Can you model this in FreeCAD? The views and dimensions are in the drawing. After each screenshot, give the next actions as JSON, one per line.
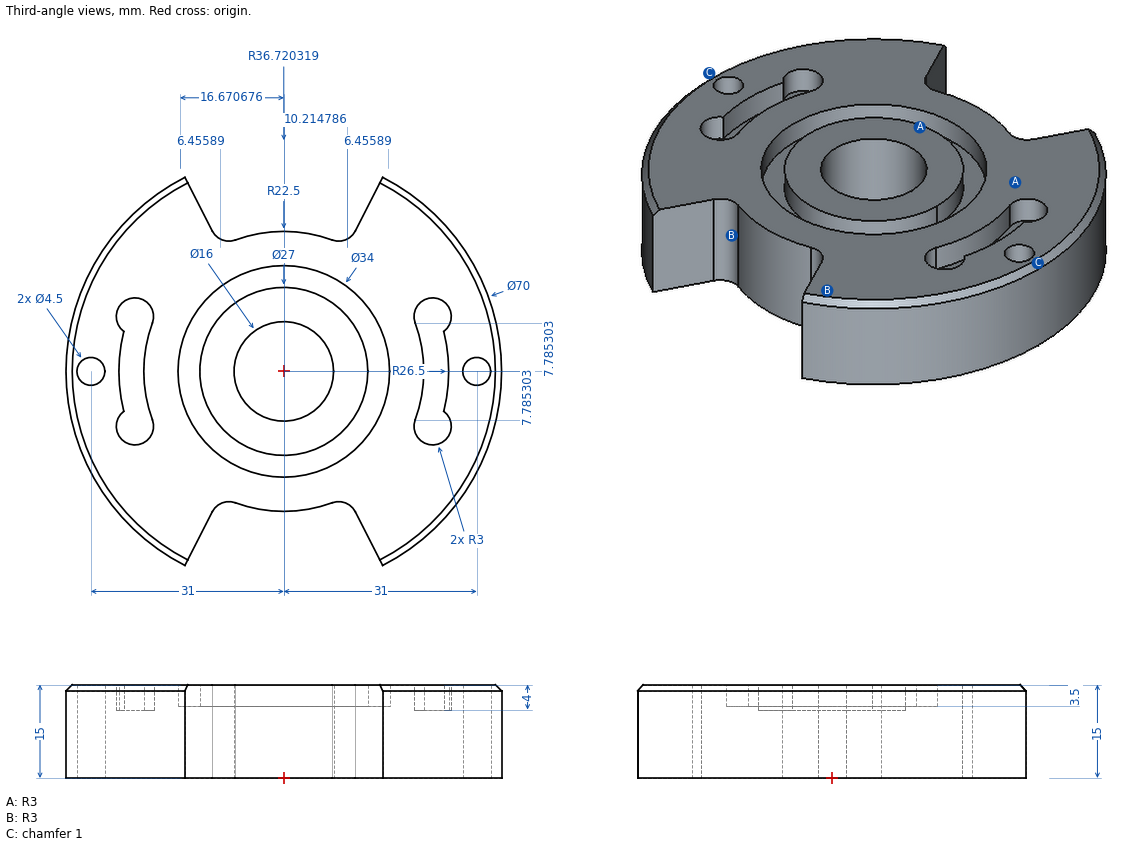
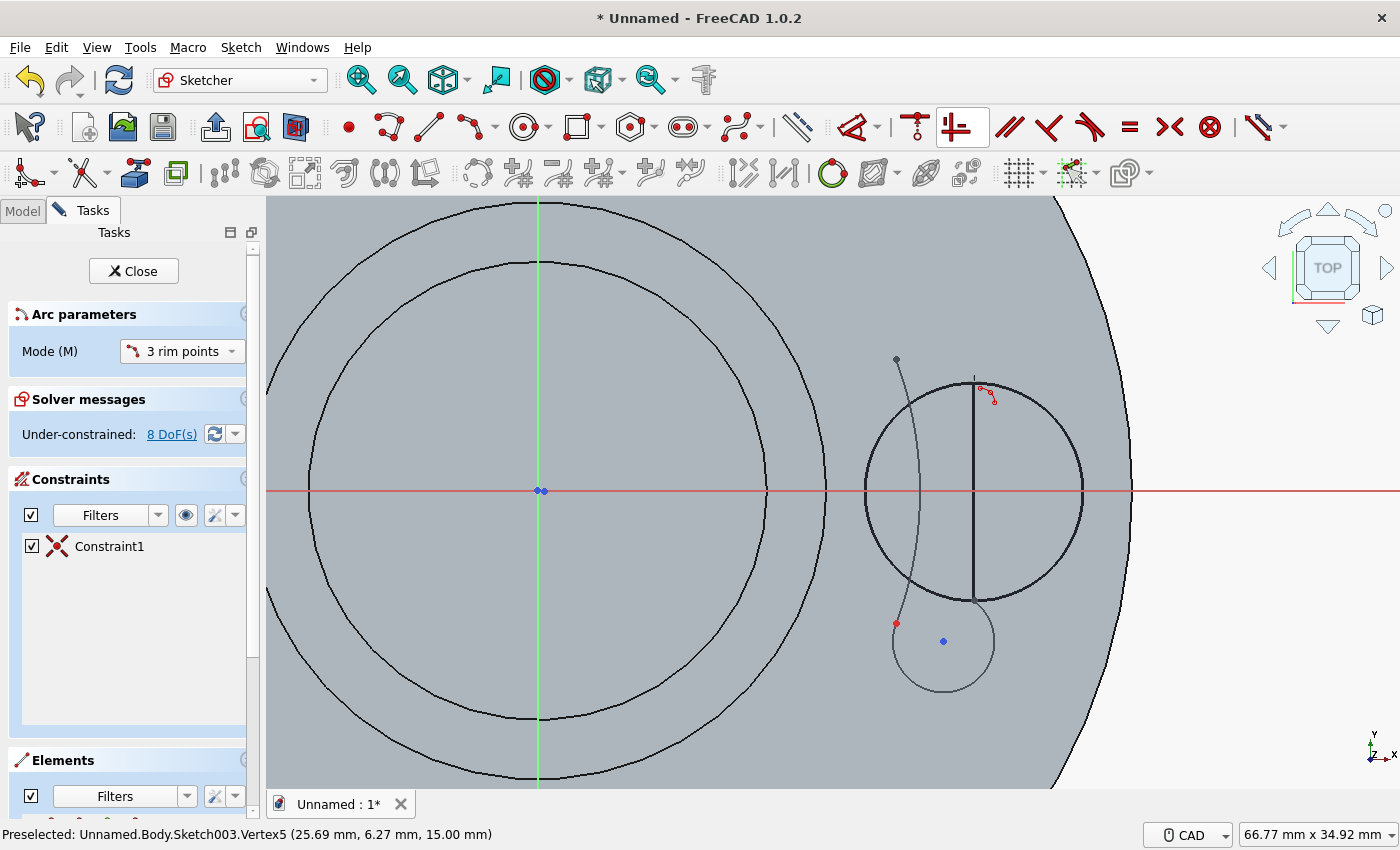
{"action": "scroll", "coordinate": [987, 513], "scroll_direction": "up", "scroll_amount": 2}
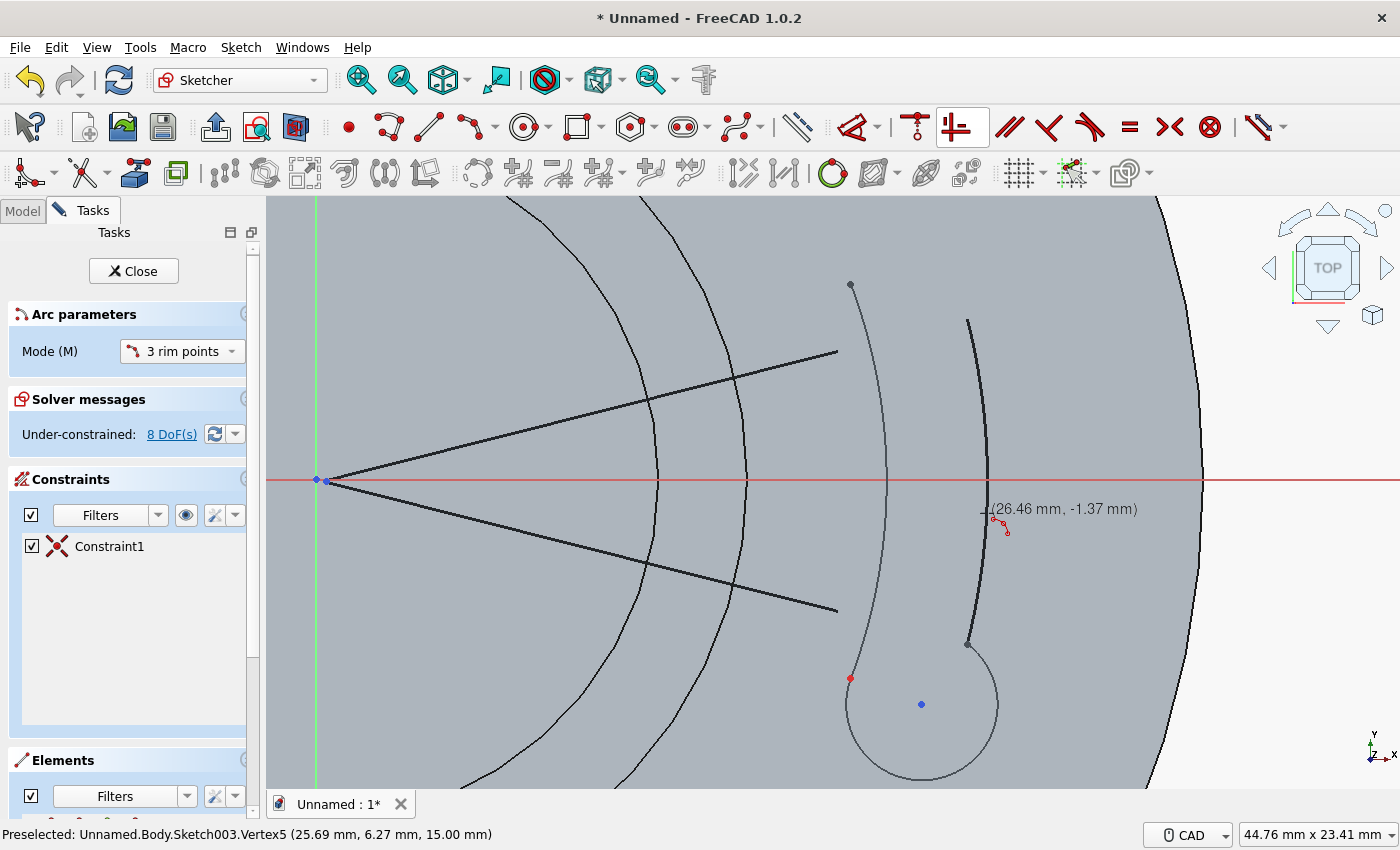
{"action": "left_click", "coordinate": [987, 512]}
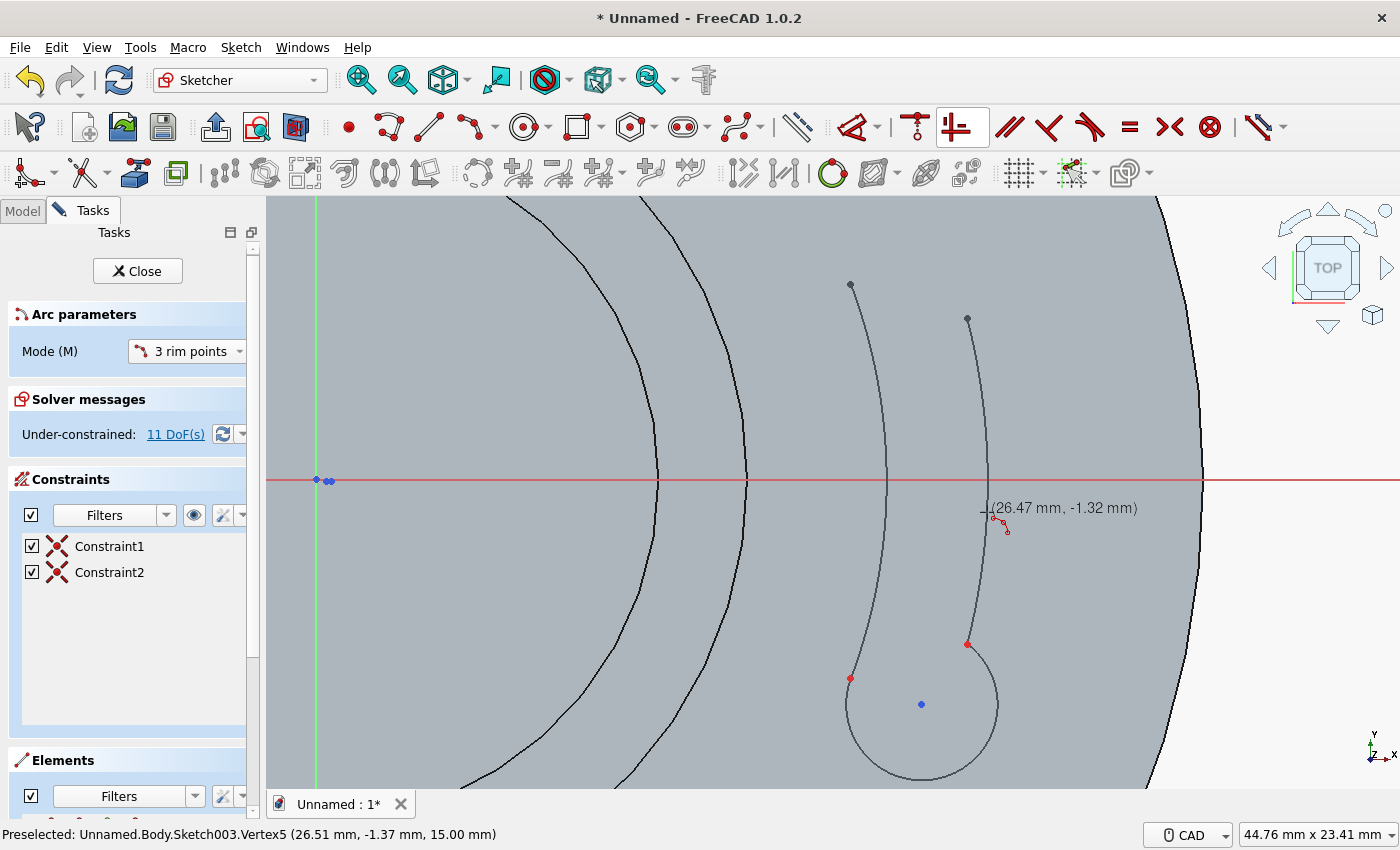
{"action": "left_click", "coordinate": [967, 319]}
{"action": "left_click", "coordinate": [851, 284]}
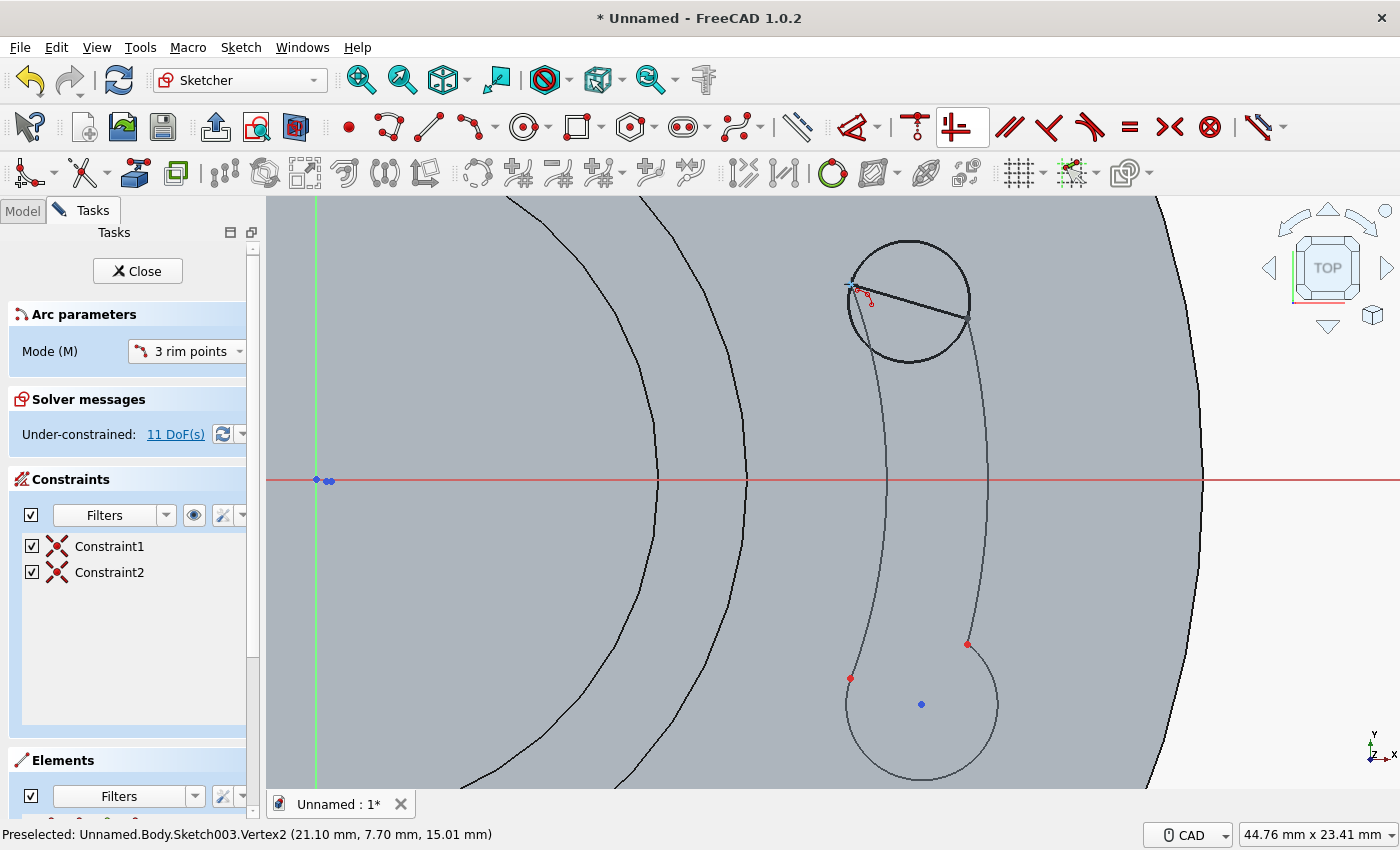
{"action": "scroll", "coordinate": [993, 519], "scroll_direction": "down", "scroll_amount": 2}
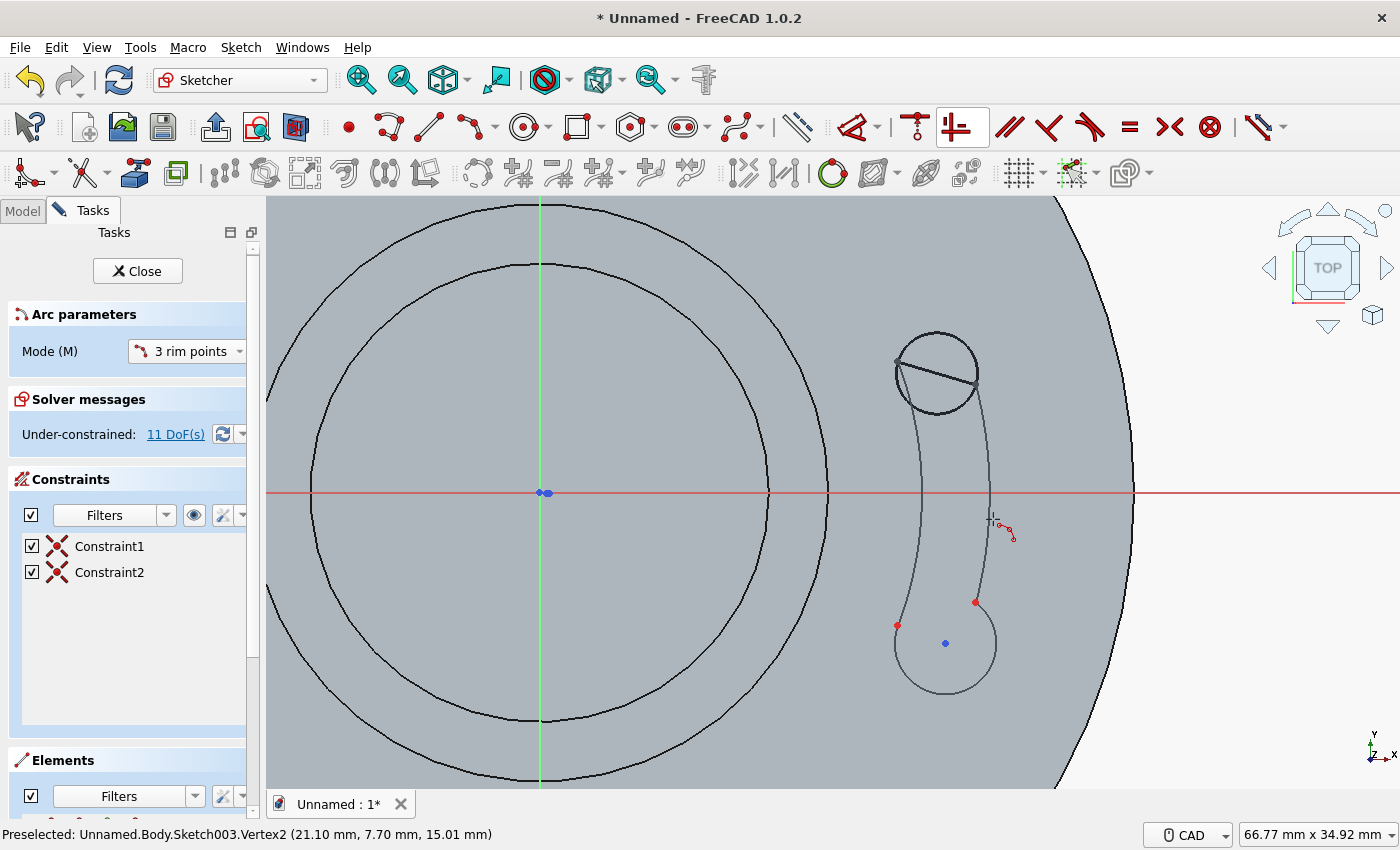
{"action": "left_click", "coordinate": [961, 294]}
{"action": "key", "text": "Escape"}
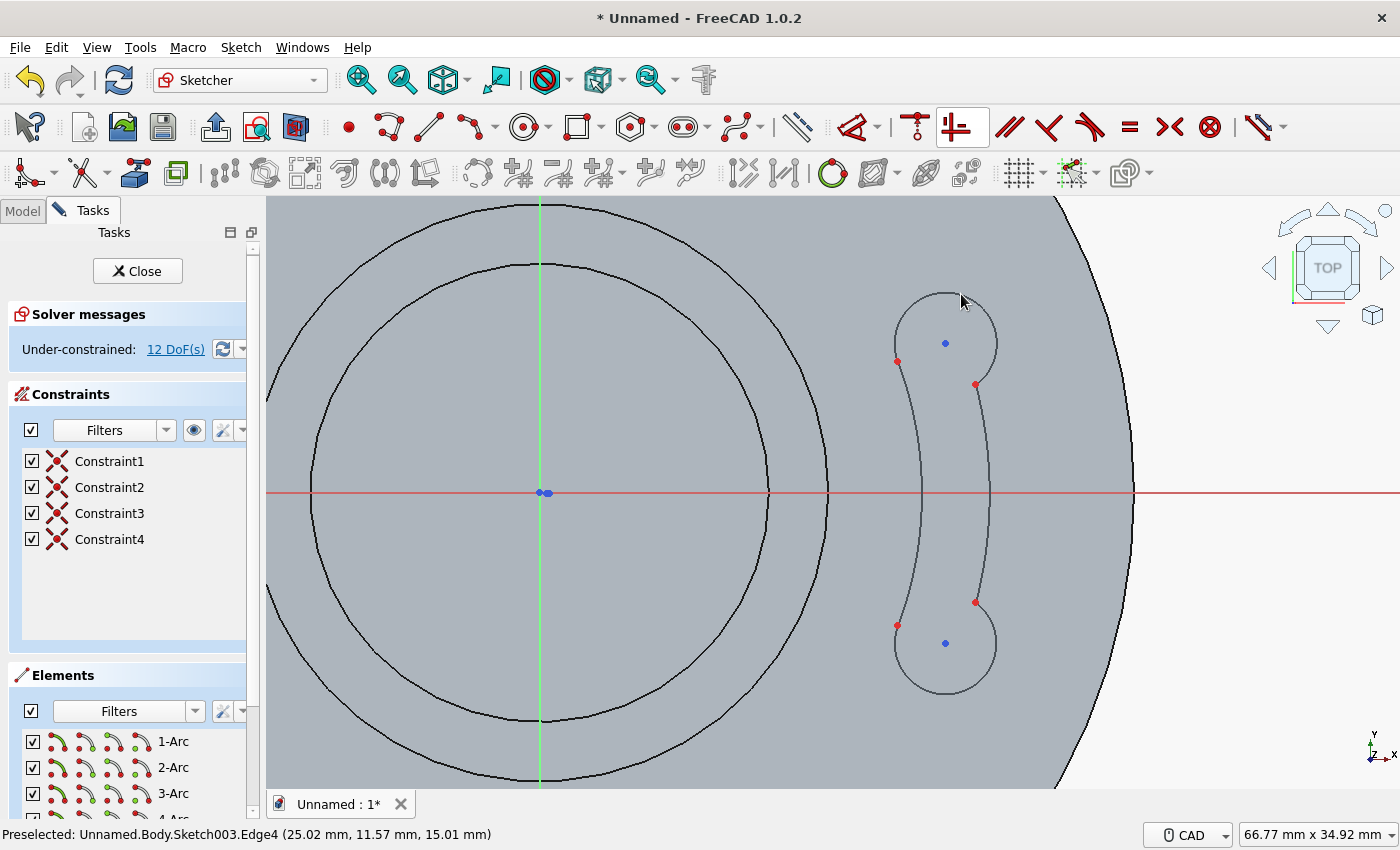
{"action": "left_click", "coordinate": [918, 548]}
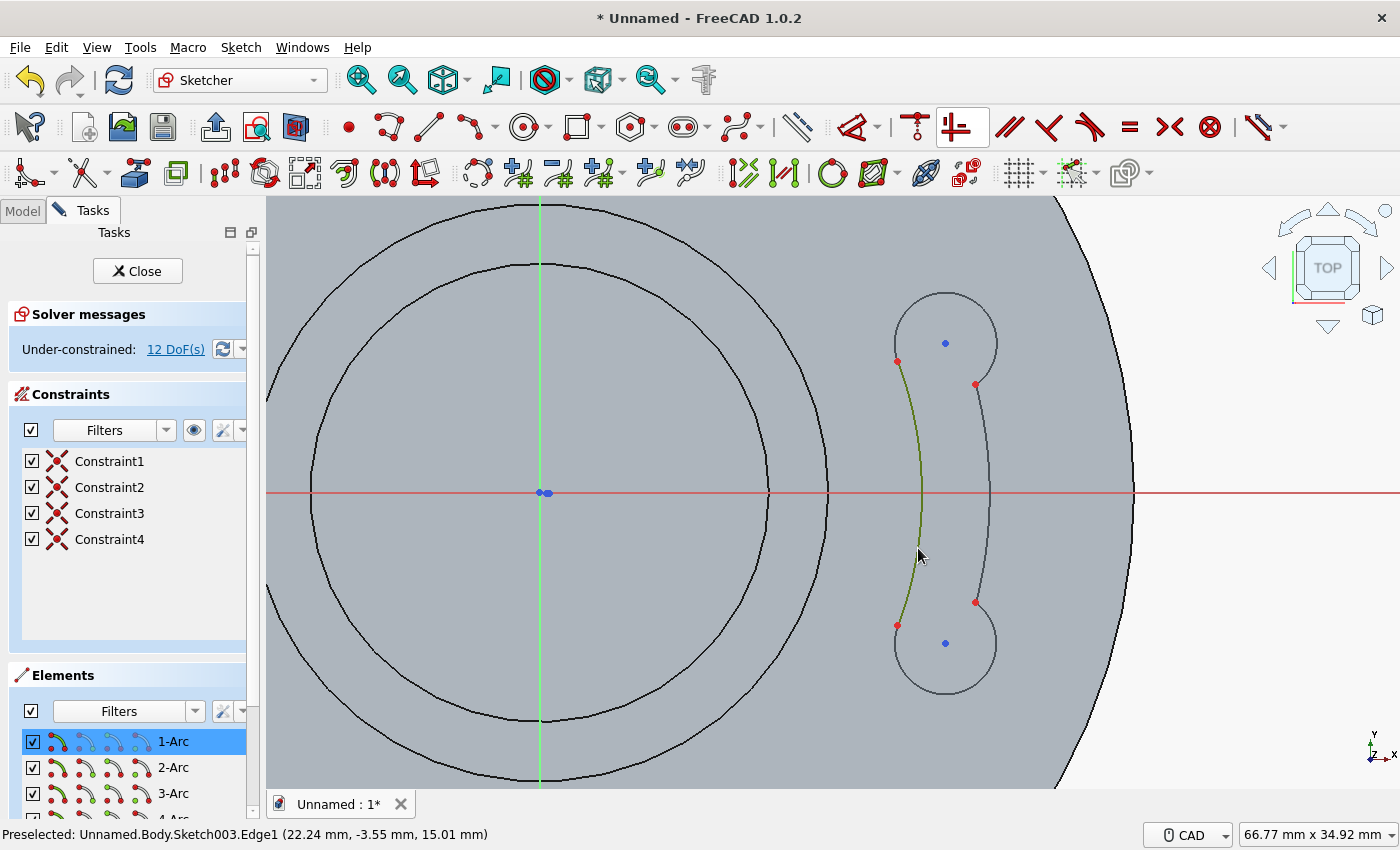
{"action": "left_click", "coordinate": [917, 686]}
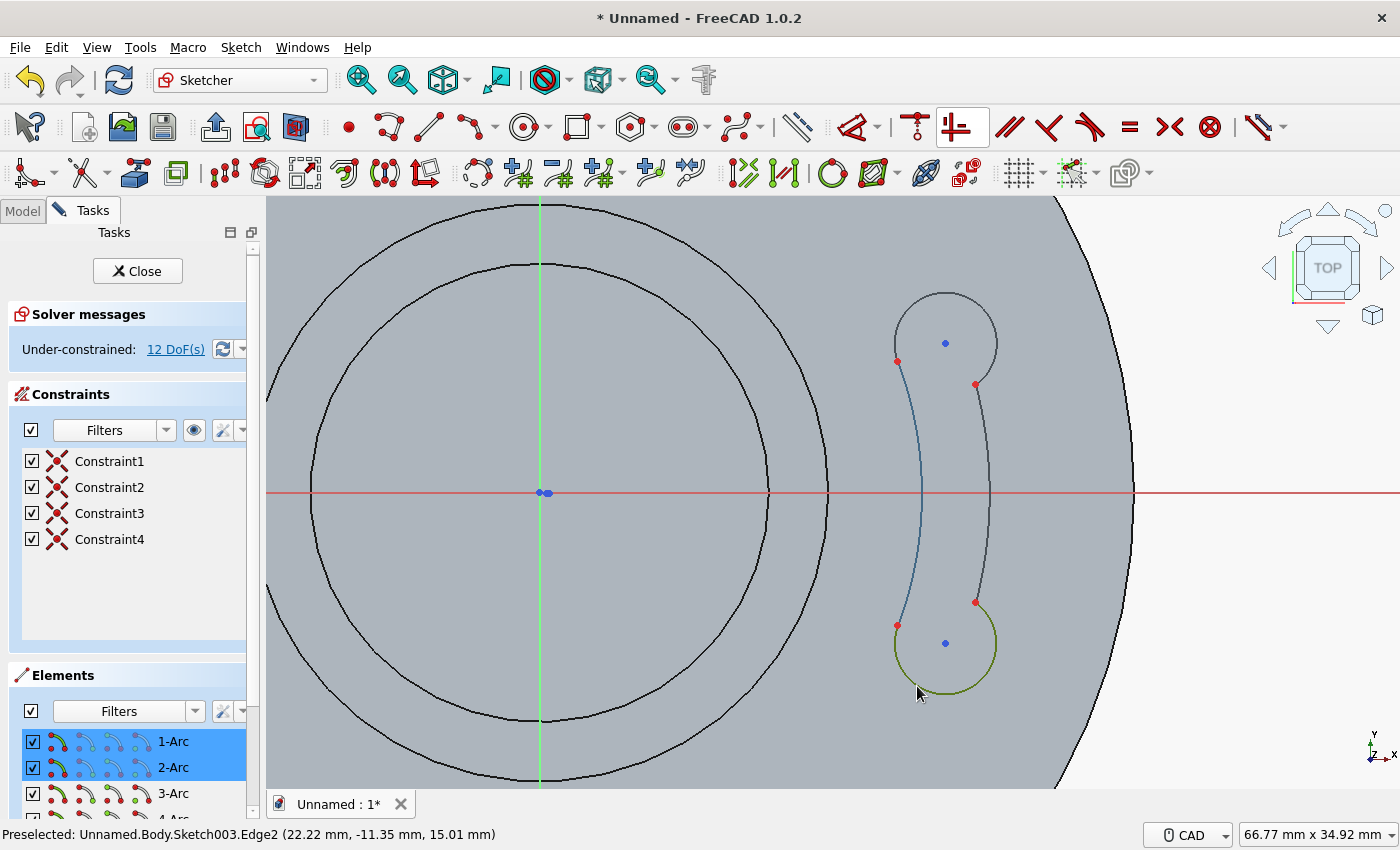
{"action": "left_click", "coordinate": [1090, 128]}